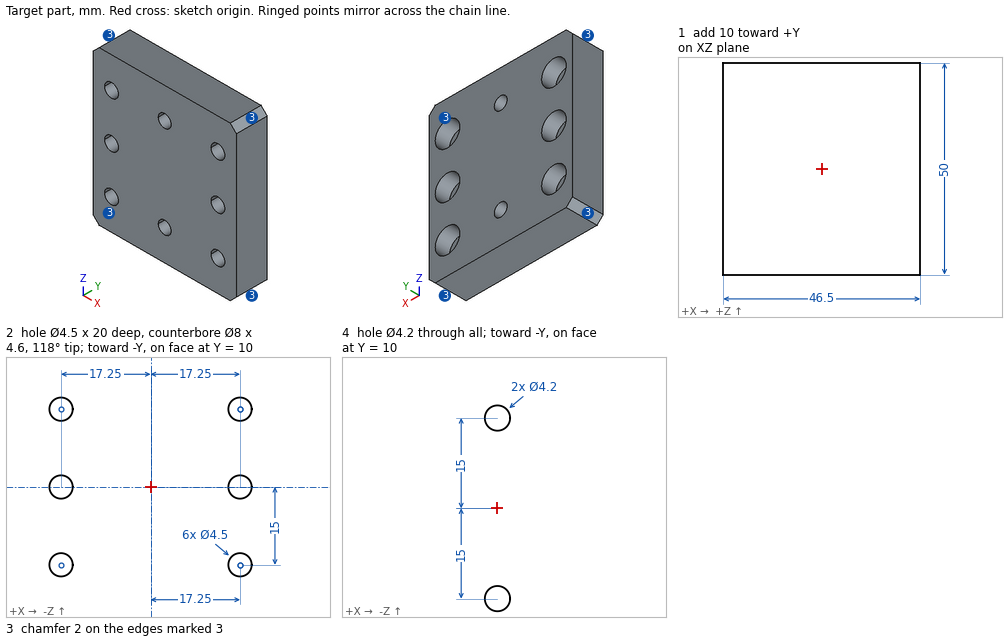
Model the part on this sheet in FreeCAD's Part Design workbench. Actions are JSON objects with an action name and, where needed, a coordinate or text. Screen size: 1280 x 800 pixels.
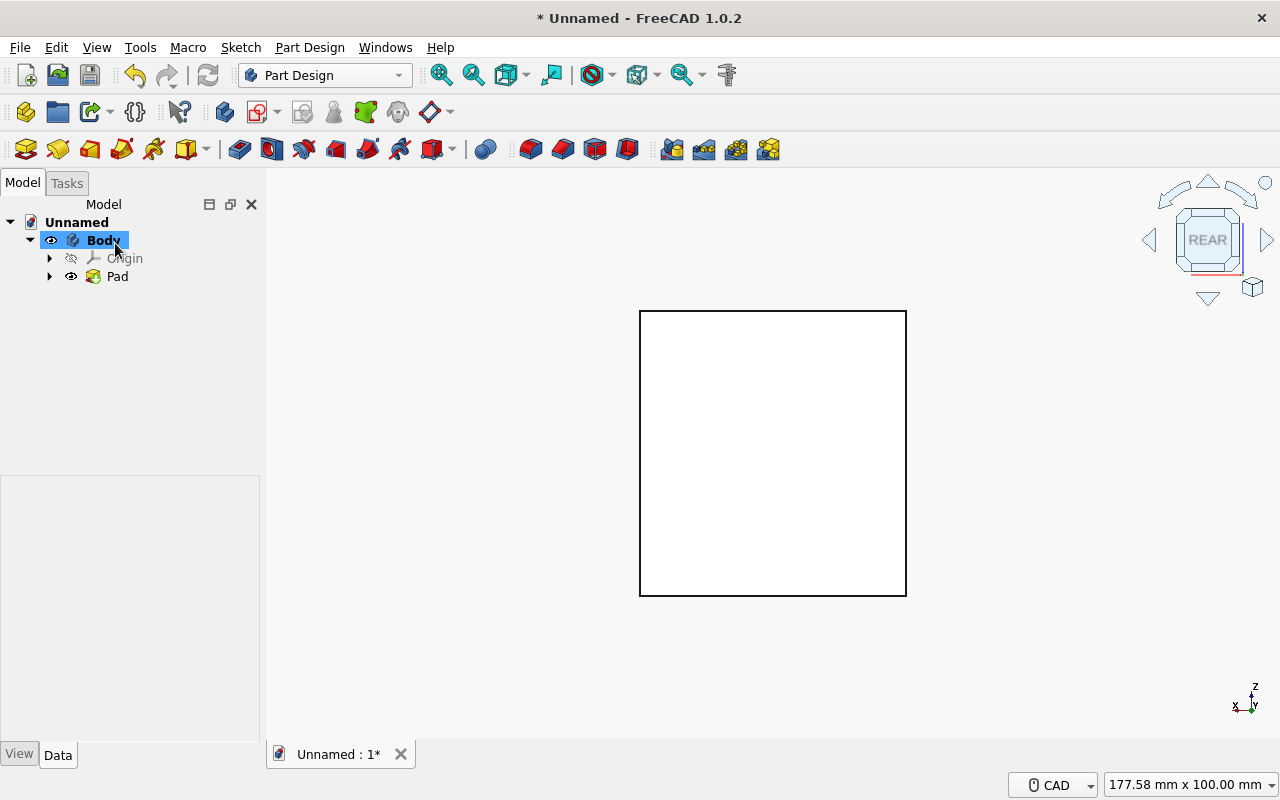
{"action": "left_click", "coordinate": [773, 452]}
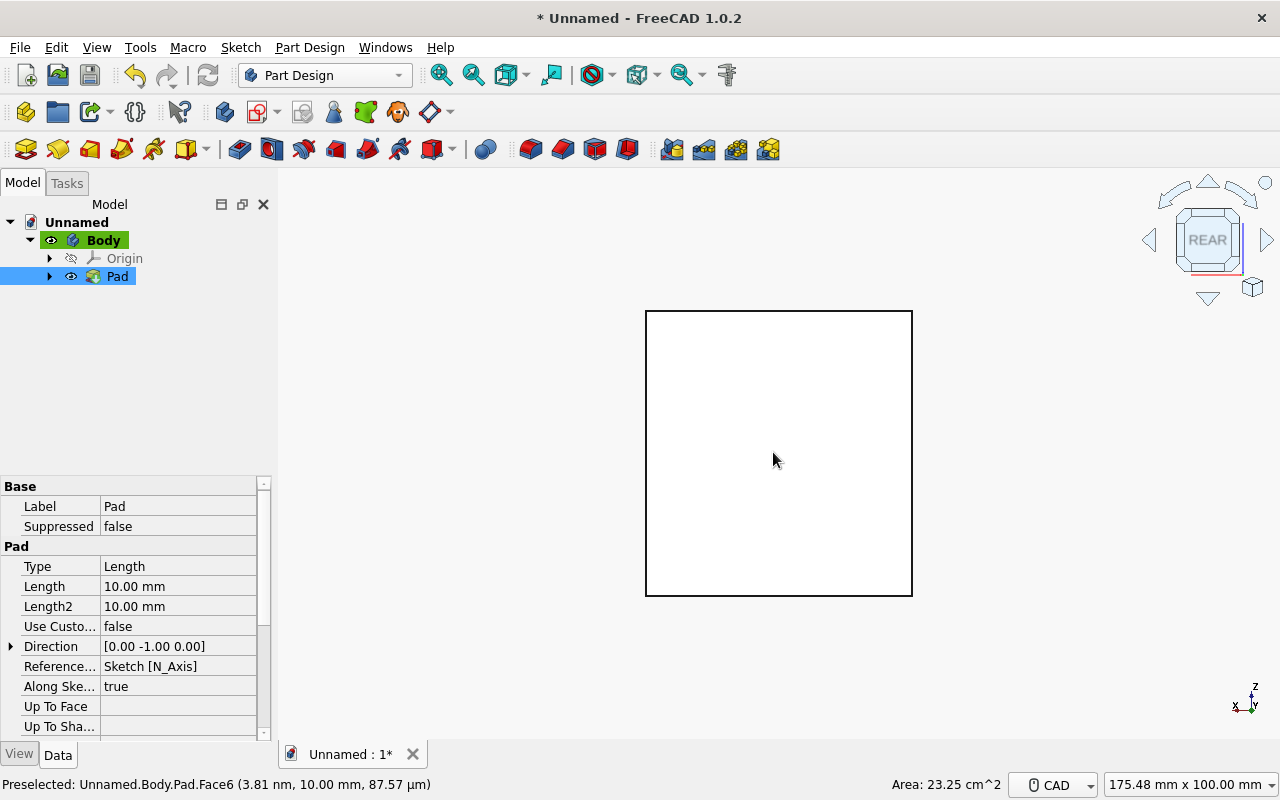
{"action": "left_click", "coordinate": [258, 112]}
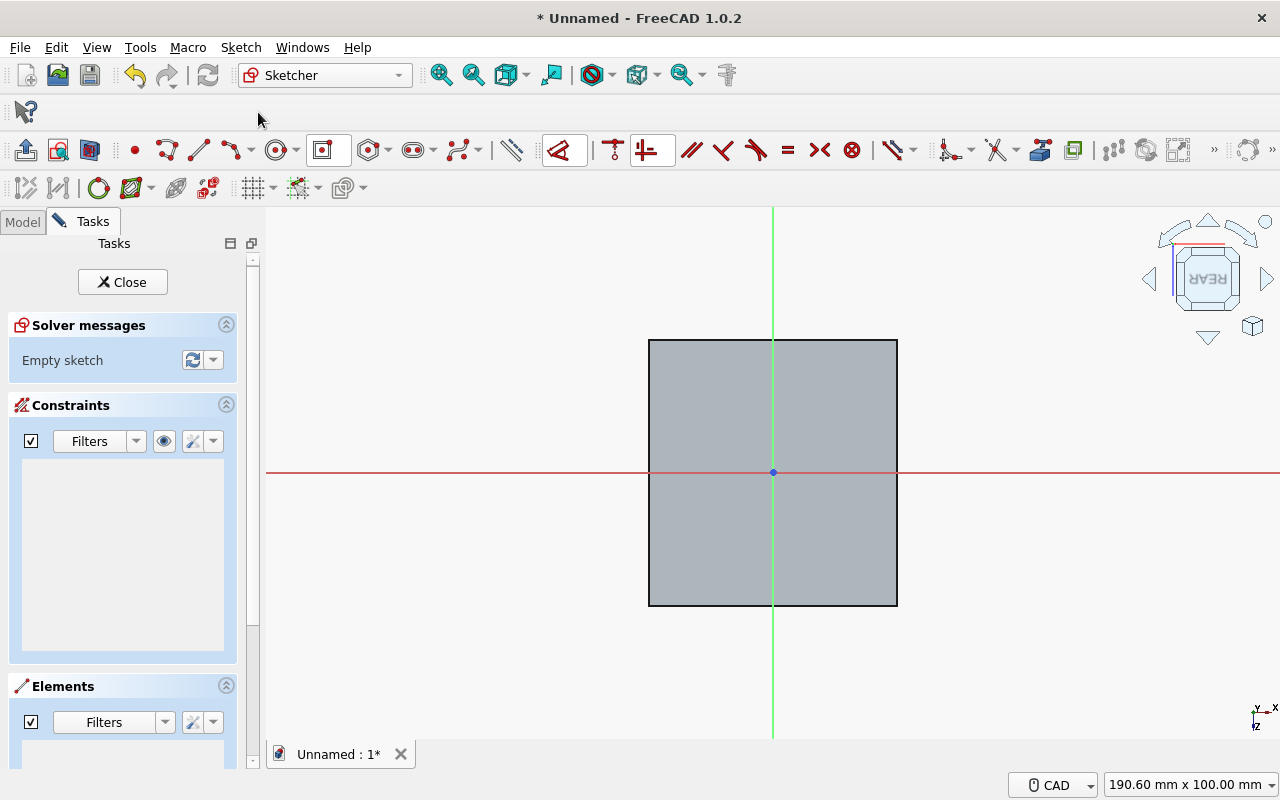
{"action": "scroll", "coordinate": [856, 473], "scroll_direction": "up", "scroll_amount": 3}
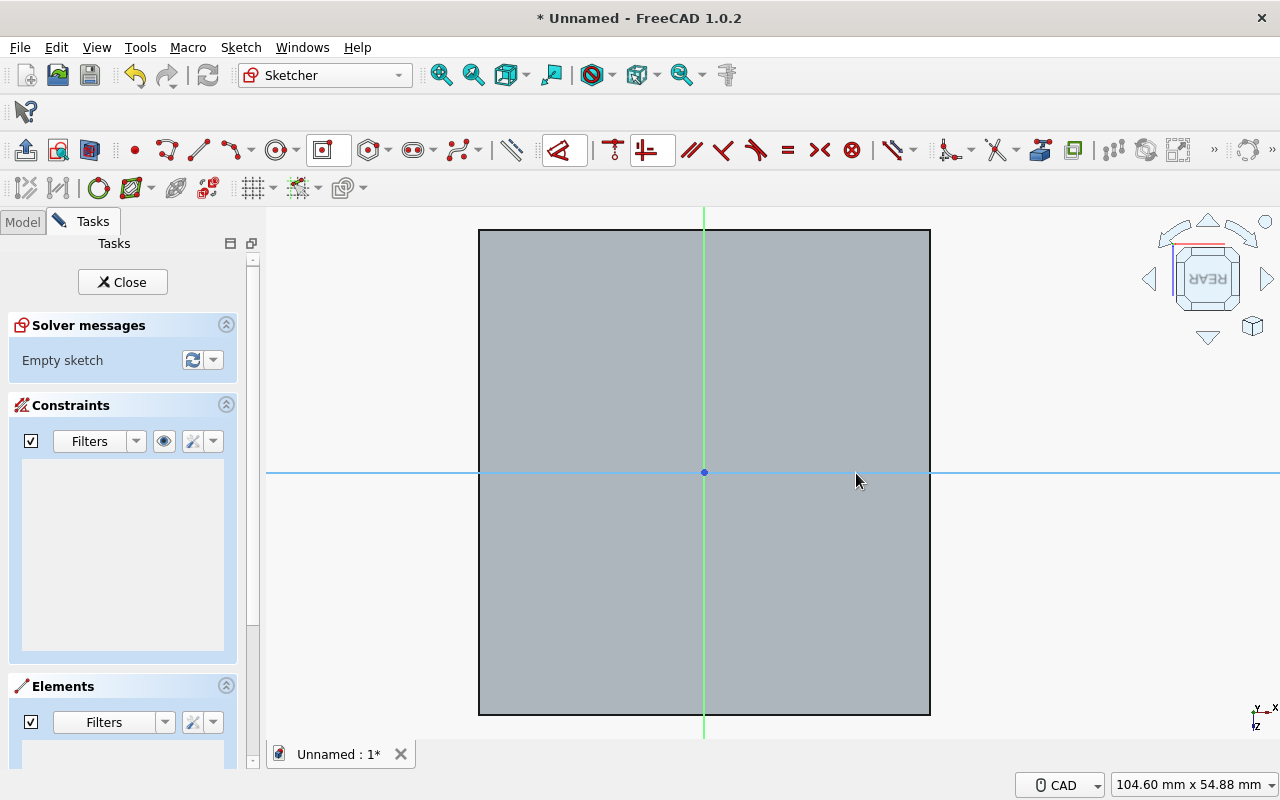
{"action": "left_click", "coordinate": [276, 150]}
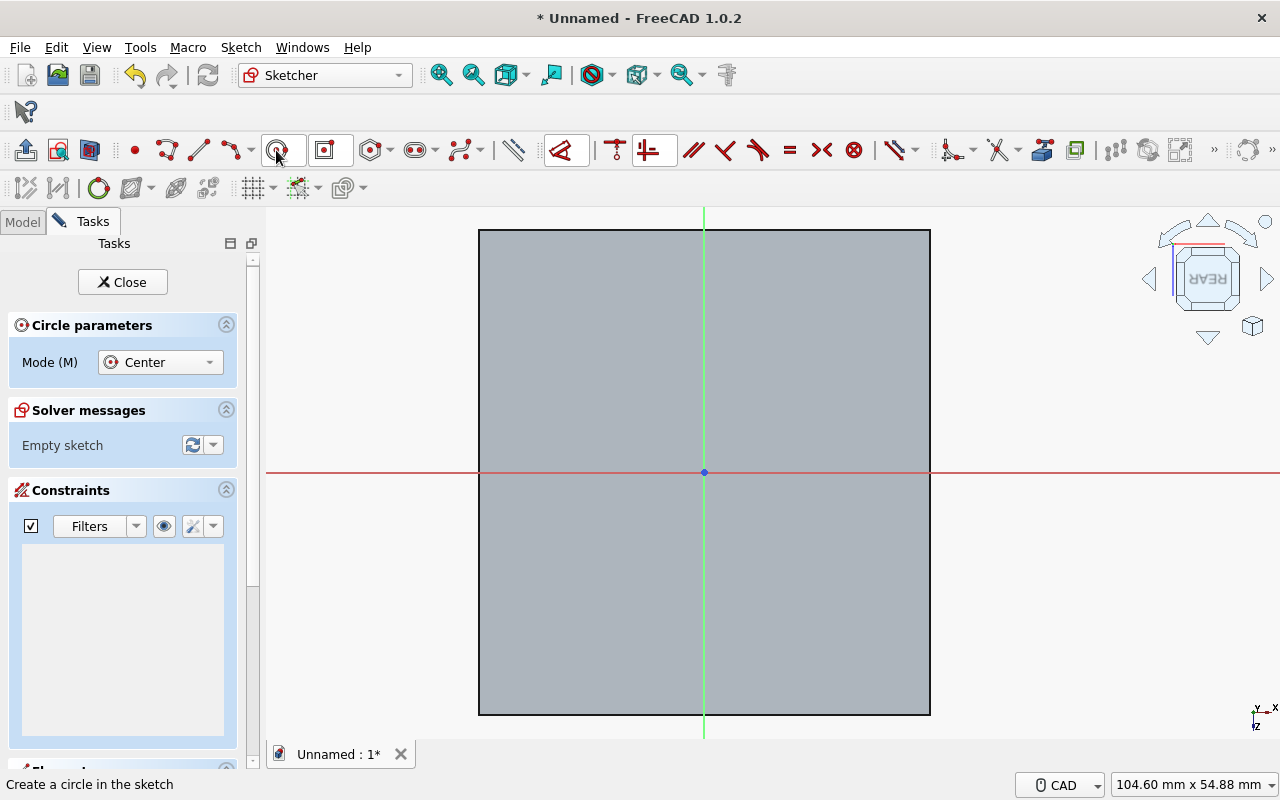
{"action": "left_click", "coordinate": [872, 618]}
{"action": "left_click", "coordinate": [887, 603]}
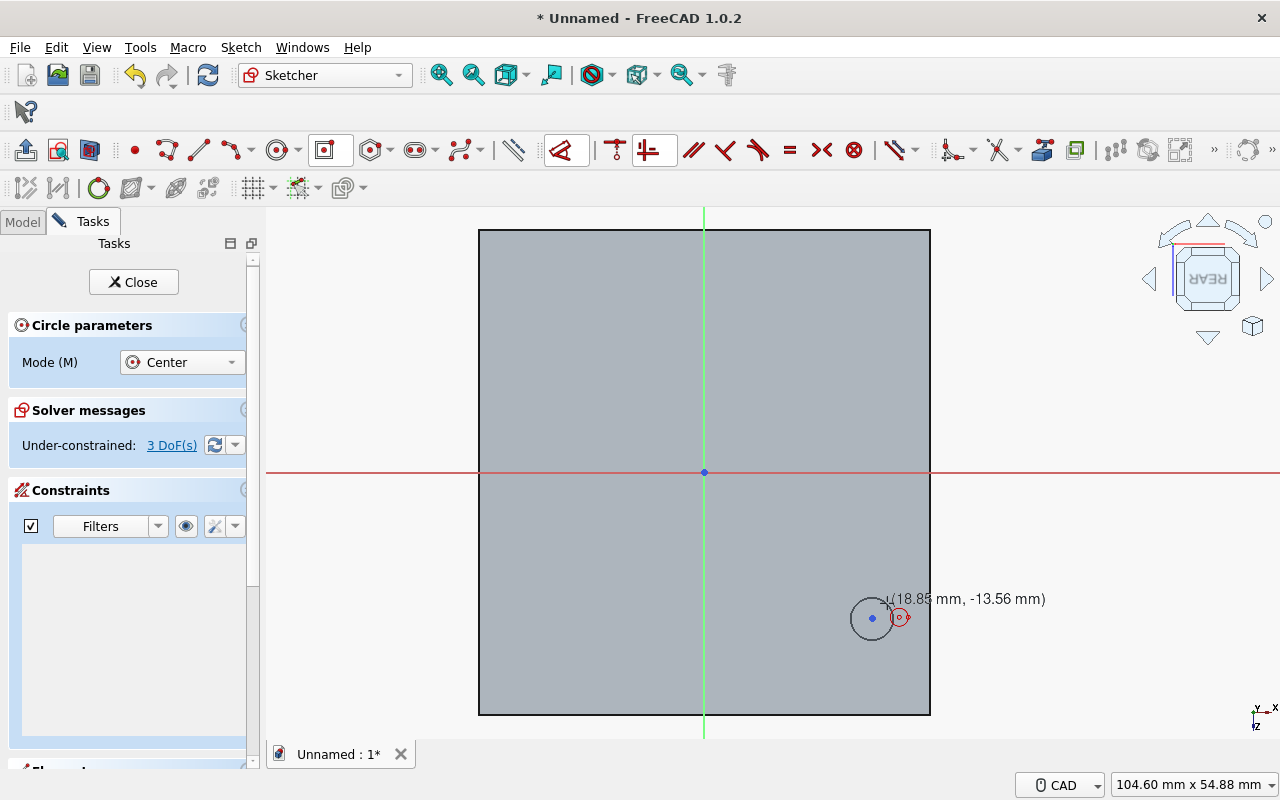
{"action": "left_click", "coordinate": [872, 473]}
{"action": "left_click", "coordinate": [887, 457]}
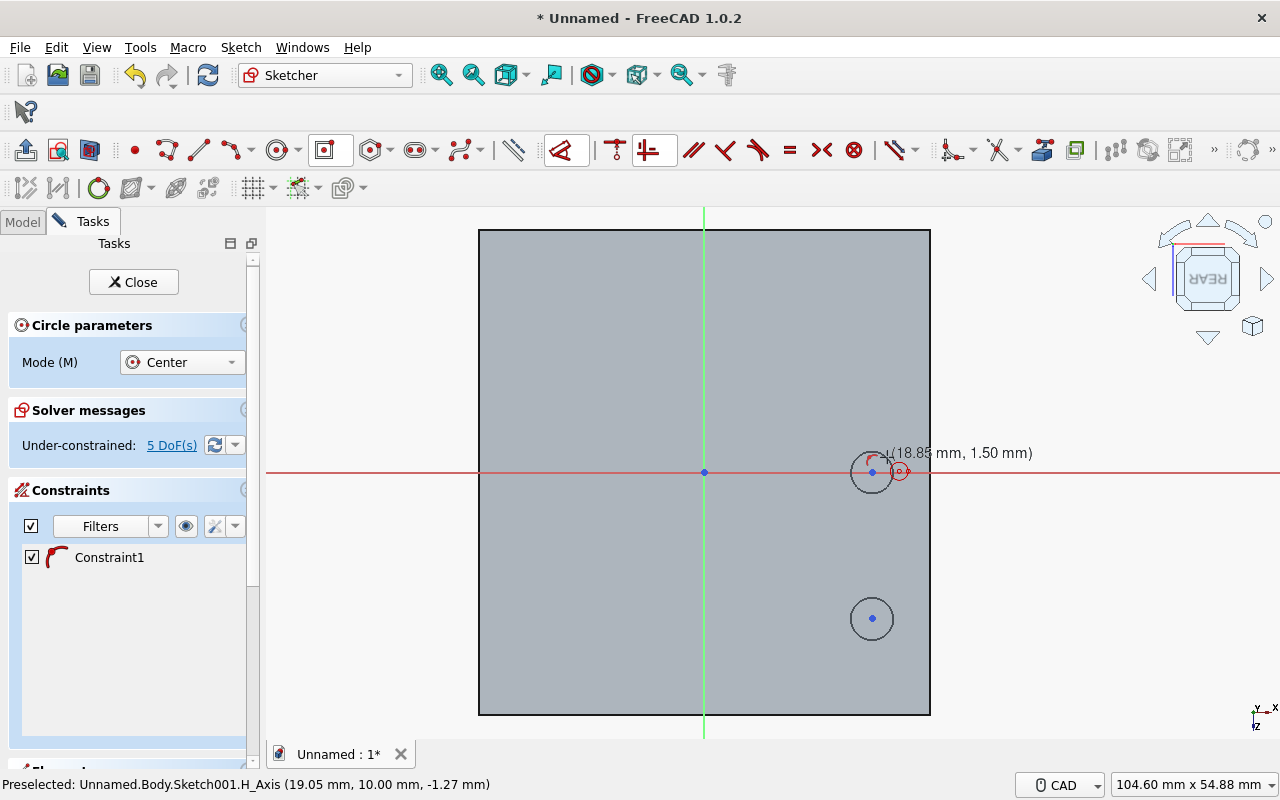
{"action": "left_click", "coordinate": [872, 327]}
{"action": "left_click", "coordinate": [887, 312]}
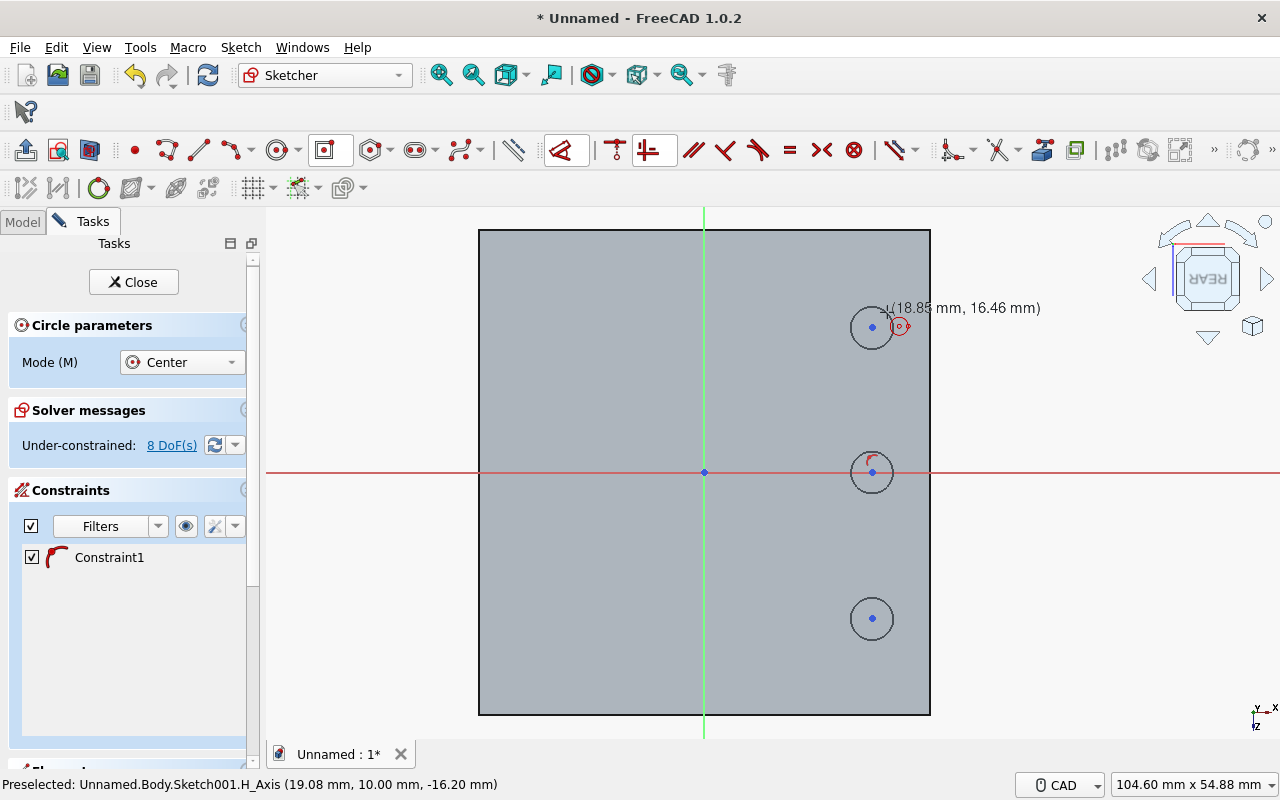
{"action": "left_click", "coordinate": [537, 327]}
{"action": "left_click", "coordinate": [552, 312]}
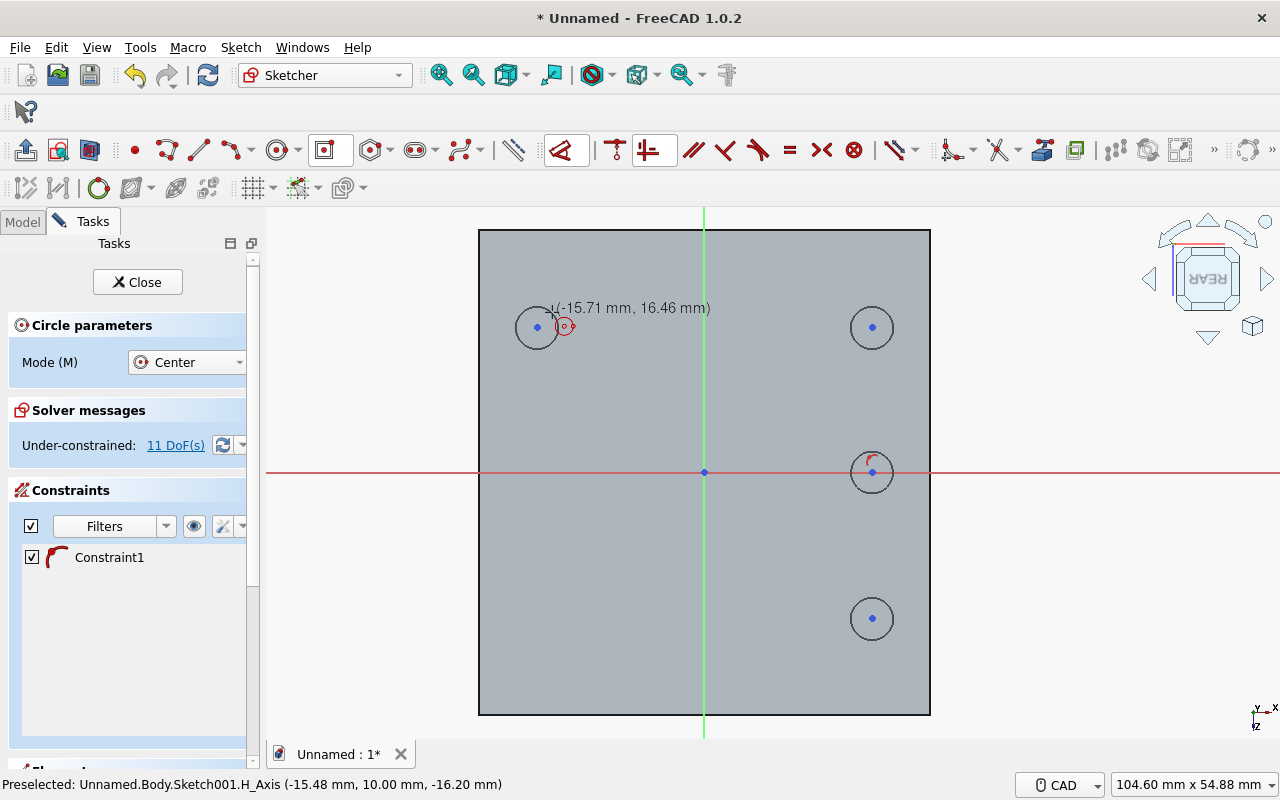
{"action": "left_click", "coordinate": [537, 473]}
{"action": "left_click", "coordinate": [552, 457]}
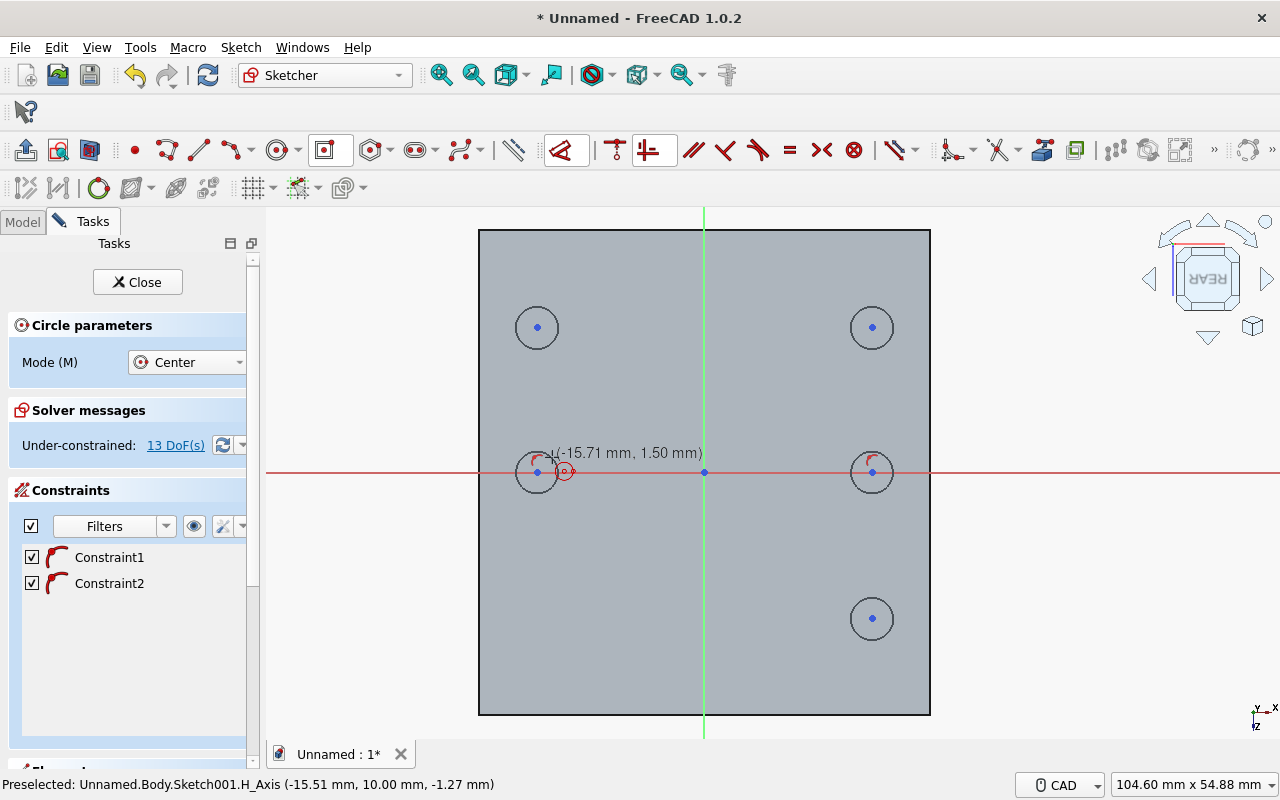
{"action": "left_click", "coordinate": [537, 618]}
{"action": "left_click", "coordinate": [552, 603]}
{"action": "key", "text": "Escape"}